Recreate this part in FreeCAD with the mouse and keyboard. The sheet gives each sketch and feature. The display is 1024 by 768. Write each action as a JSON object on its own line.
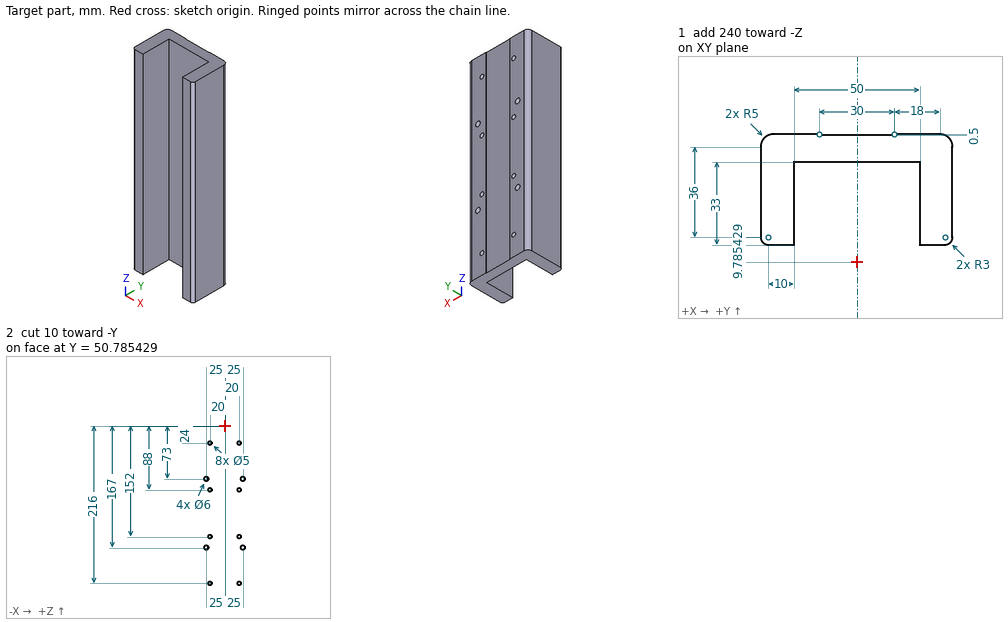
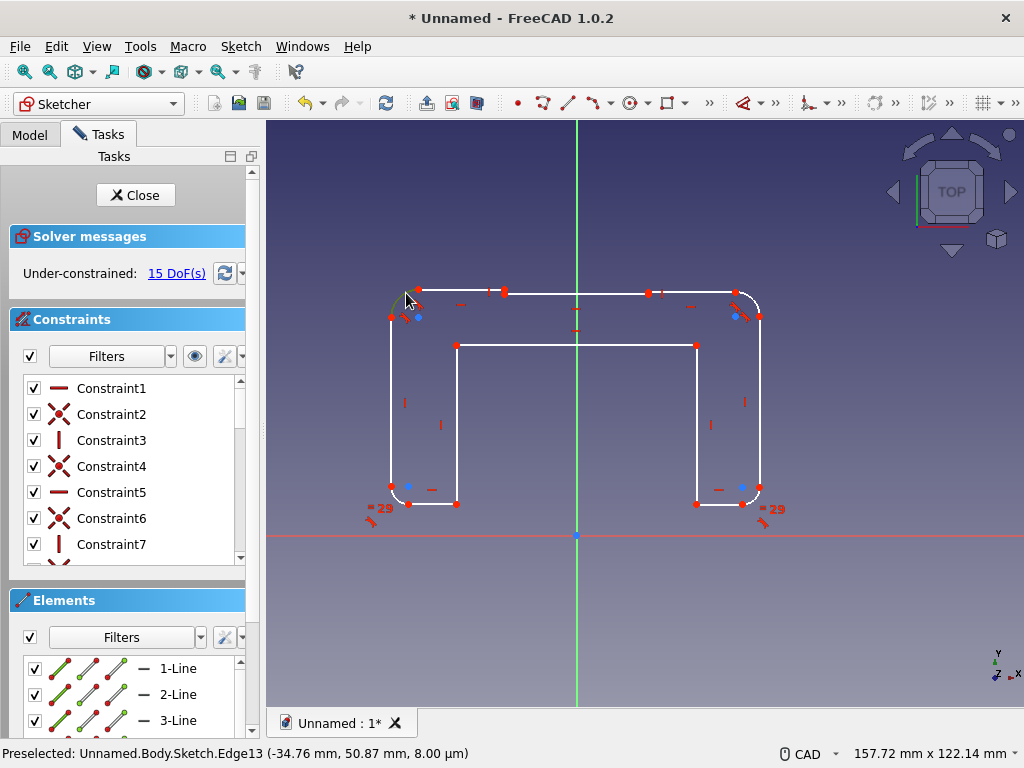
{"action": "left_click", "coordinate": [757, 305]}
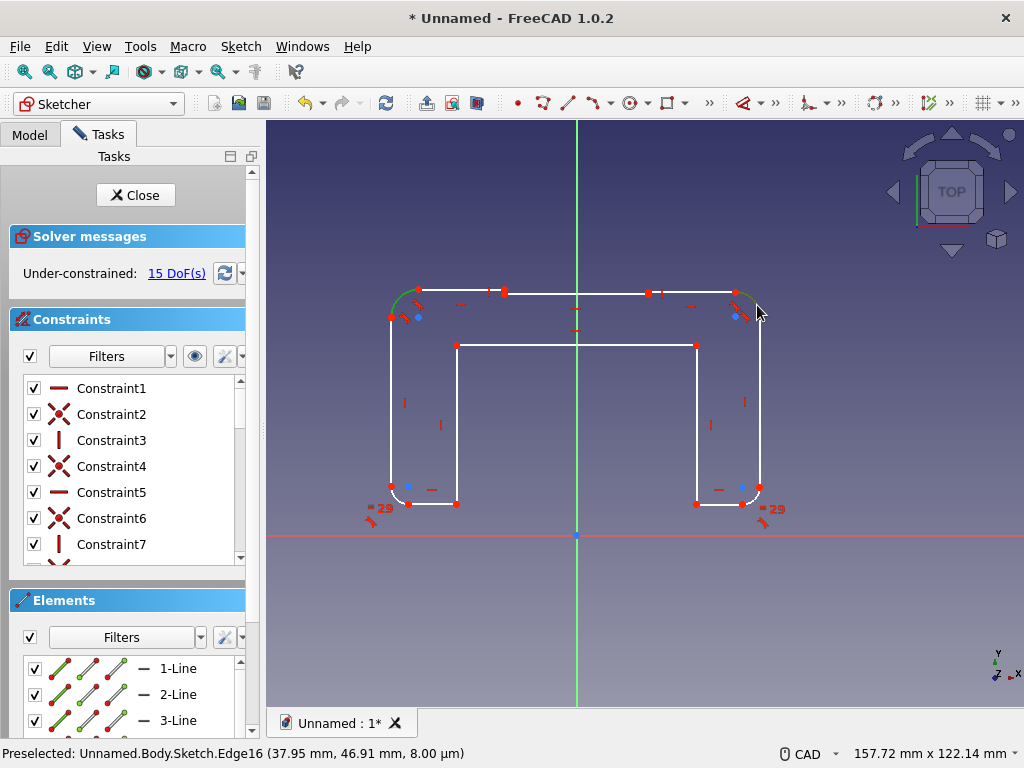
{"action": "key", "text": "e"}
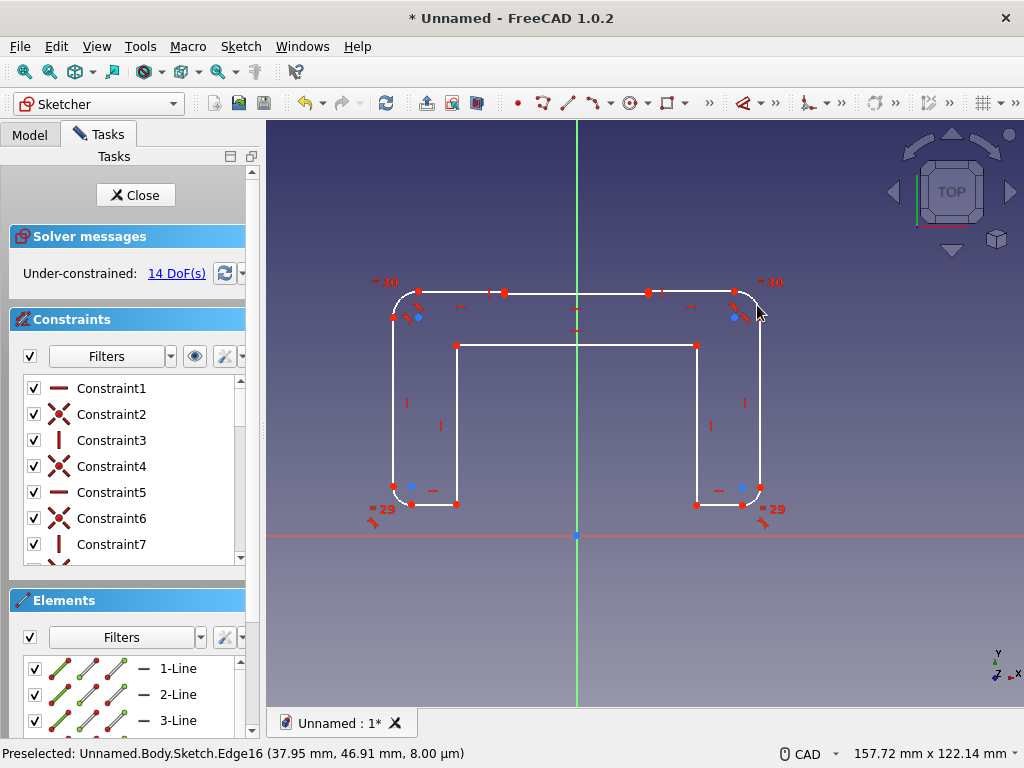
{"action": "left_click", "coordinate": [411, 487]}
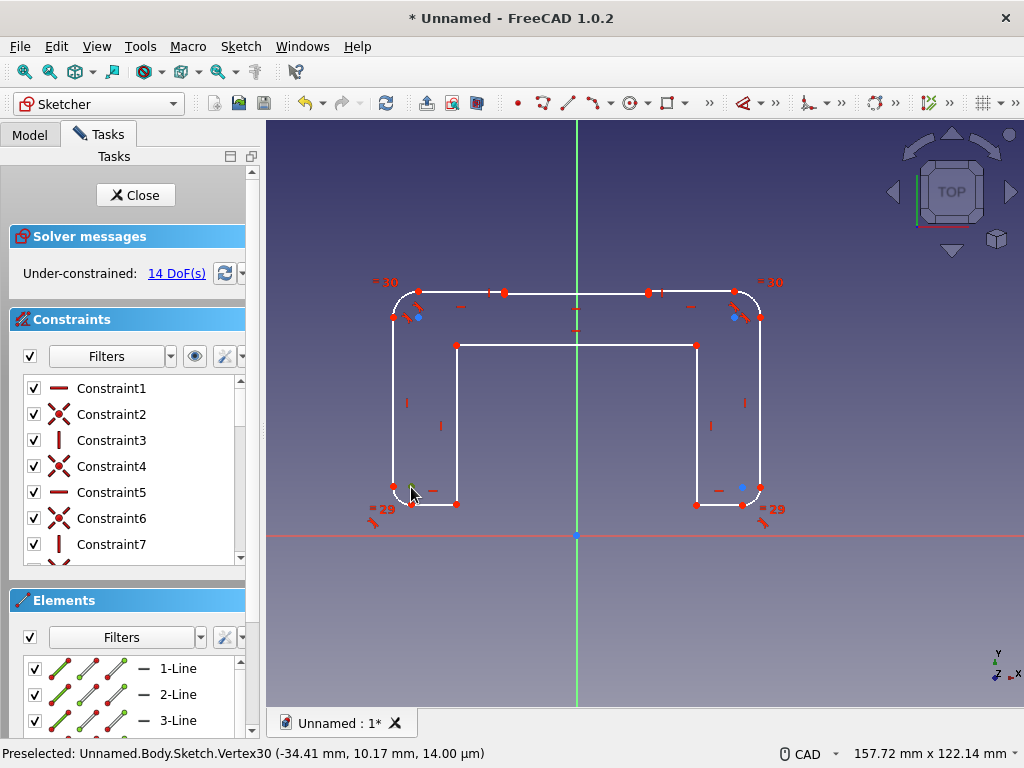
{"action": "left_click", "coordinate": [742, 487]}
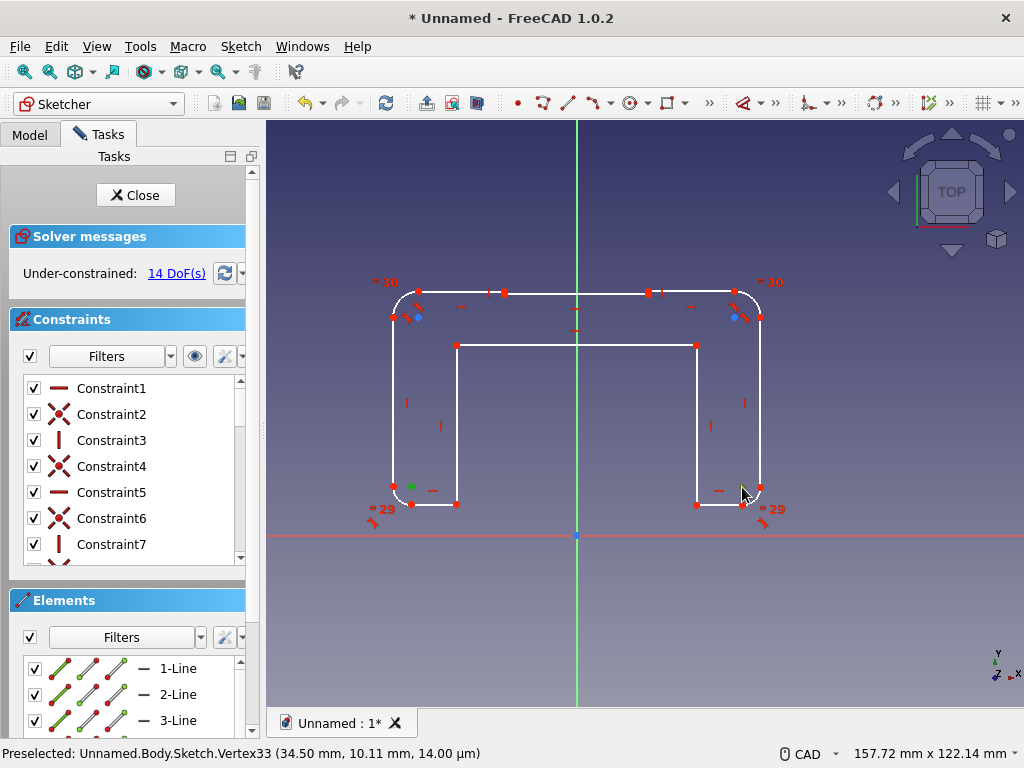
{"action": "left_click", "coordinate": [577, 641]}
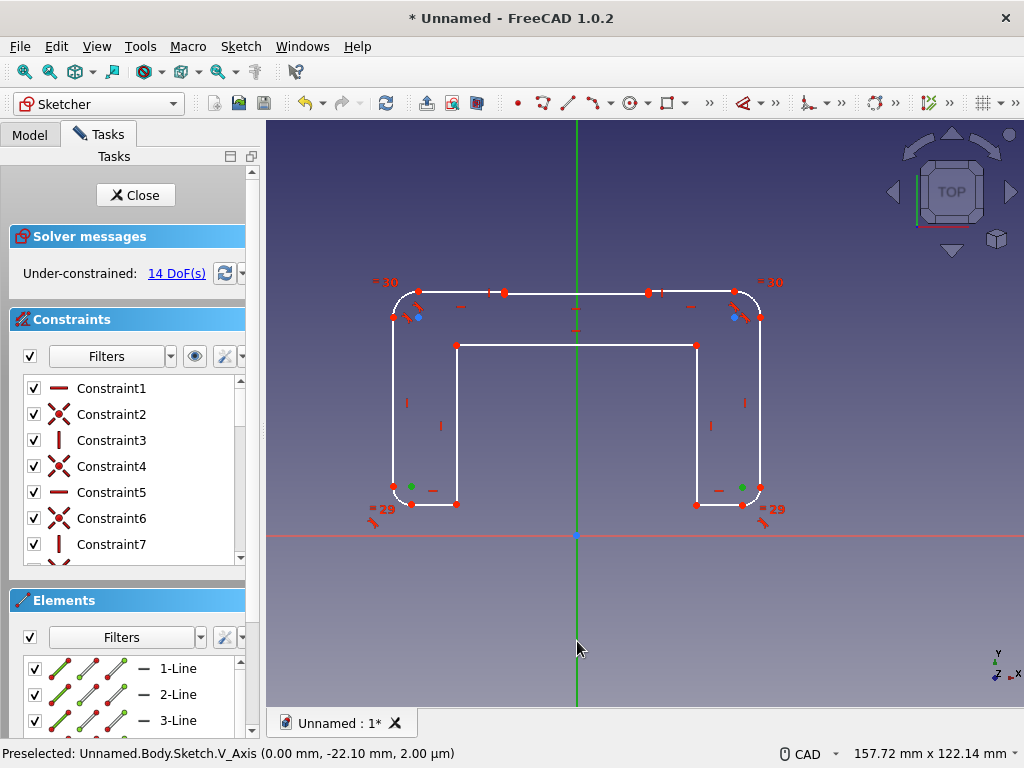
{"action": "key", "text": "s"}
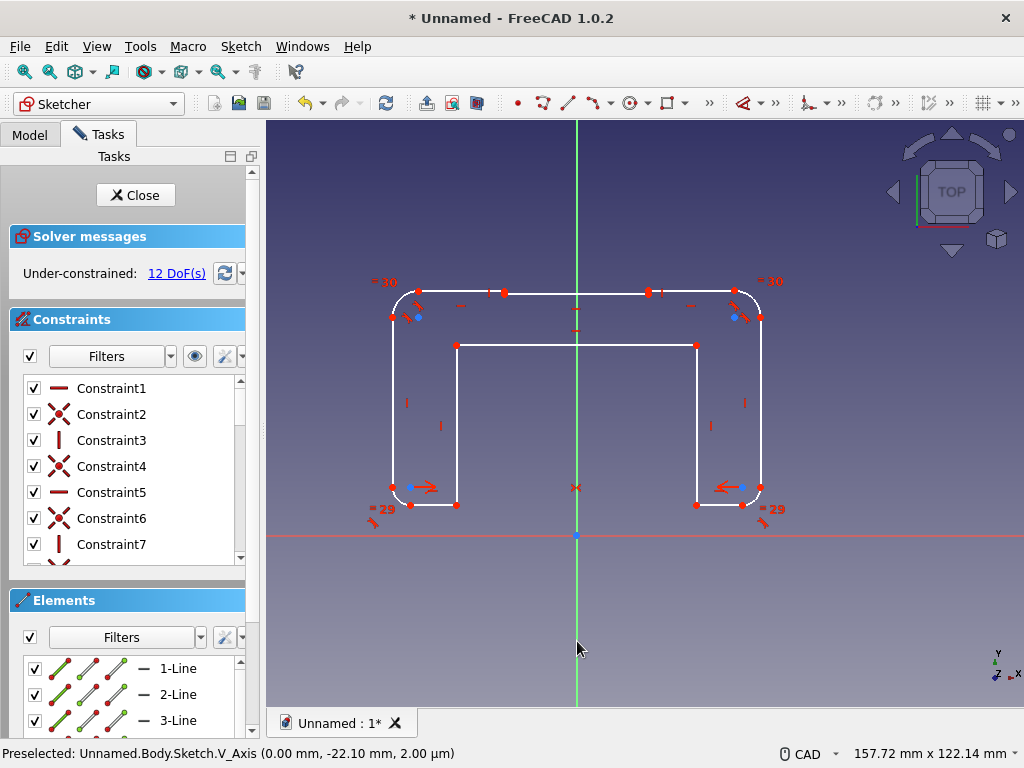
{"action": "scroll", "coordinate": [648, 291], "scroll_direction": "up", "scroll_amount": 7}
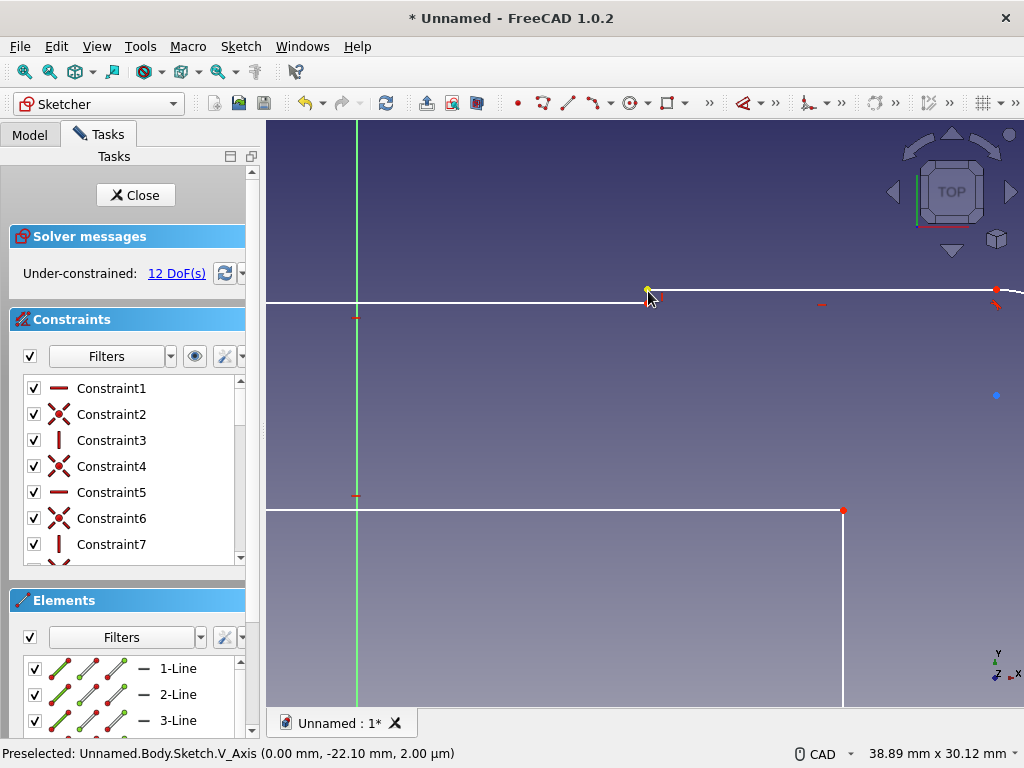
{"action": "left_click", "coordinate": [648, 290]}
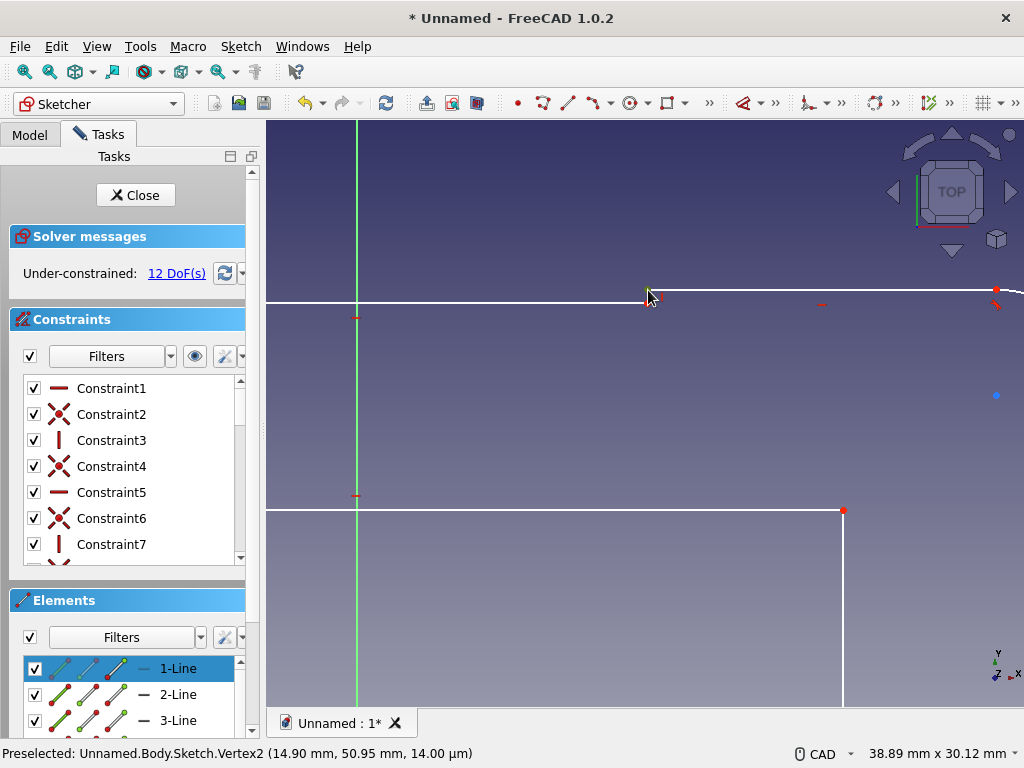
{"action": "scroll", "coordinate": [648, 291], "scroll_direction": "down", "scroll_amount": 7}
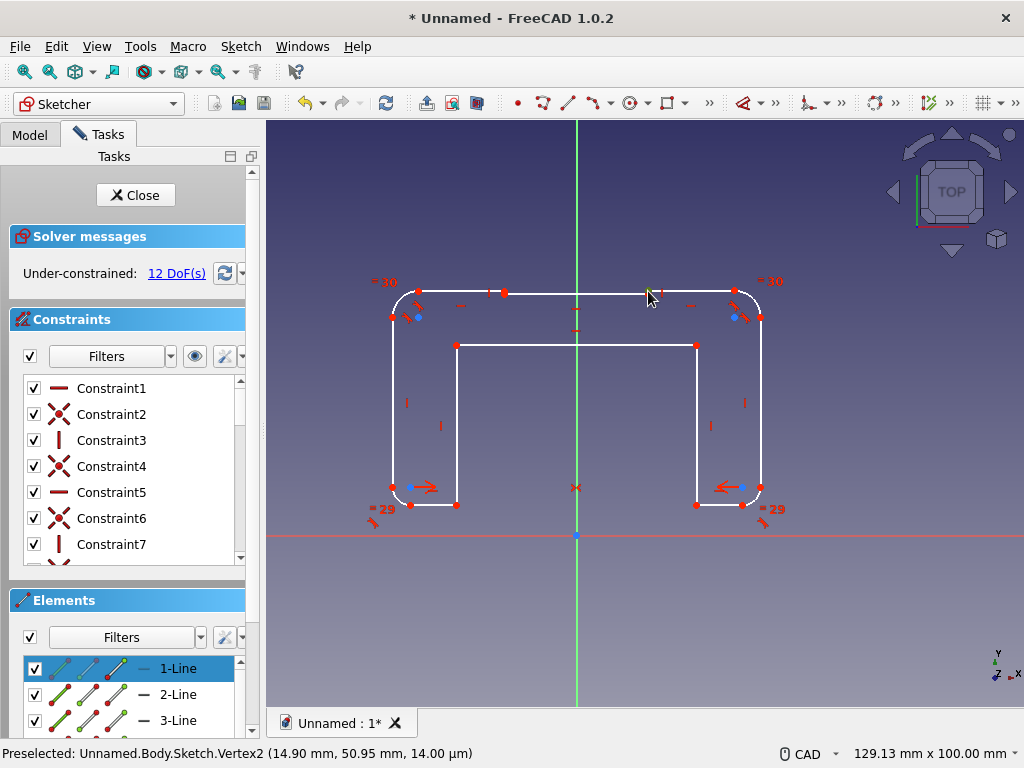
{"action": "scroll", "coordinate": [505, 291], "scroll_direction": "up", "scroll_amount": 7}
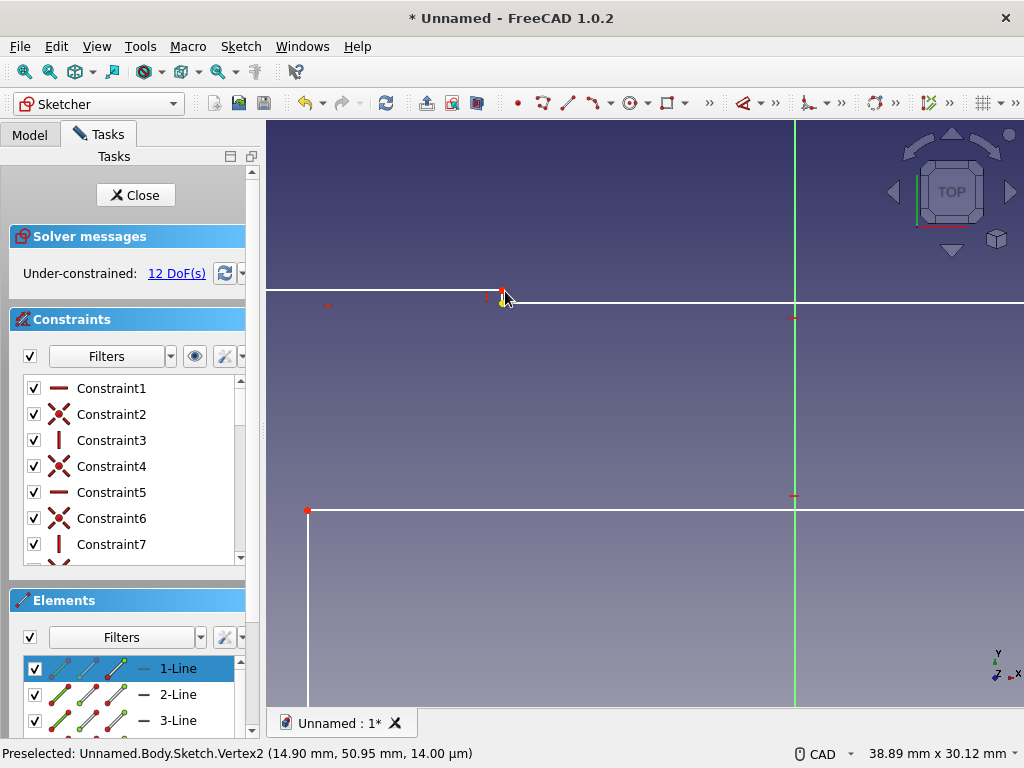
{"action": "left_click", "coordinate": [502, 290]}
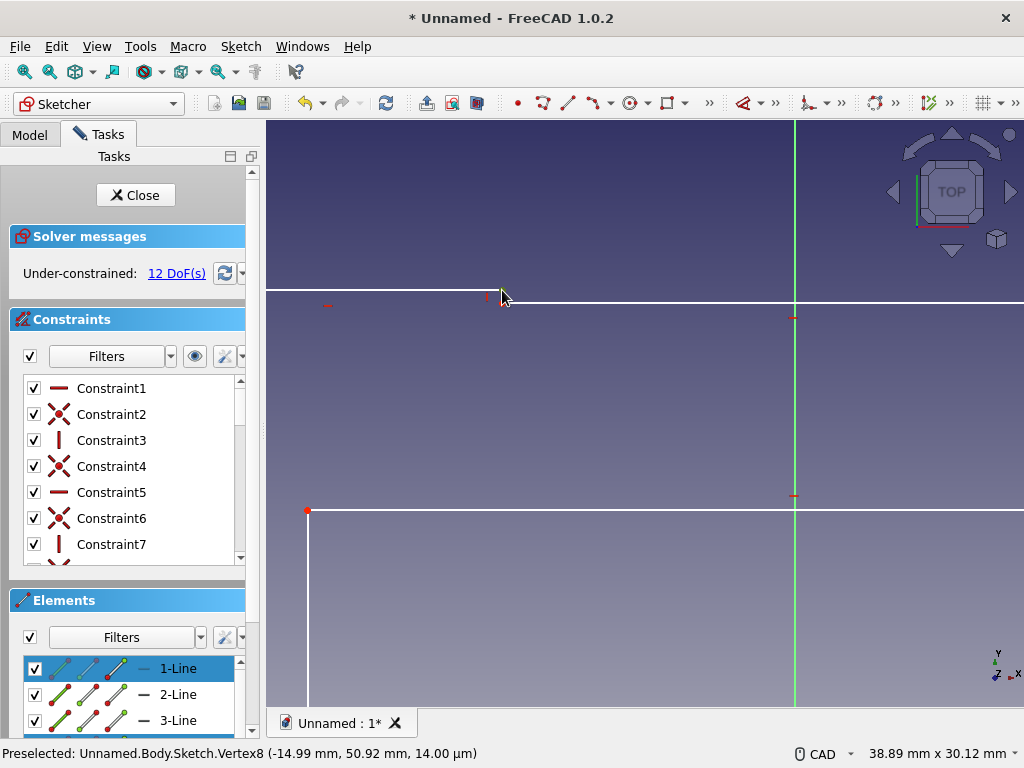
{"action": "left_click", "coordinate": [795, 641]}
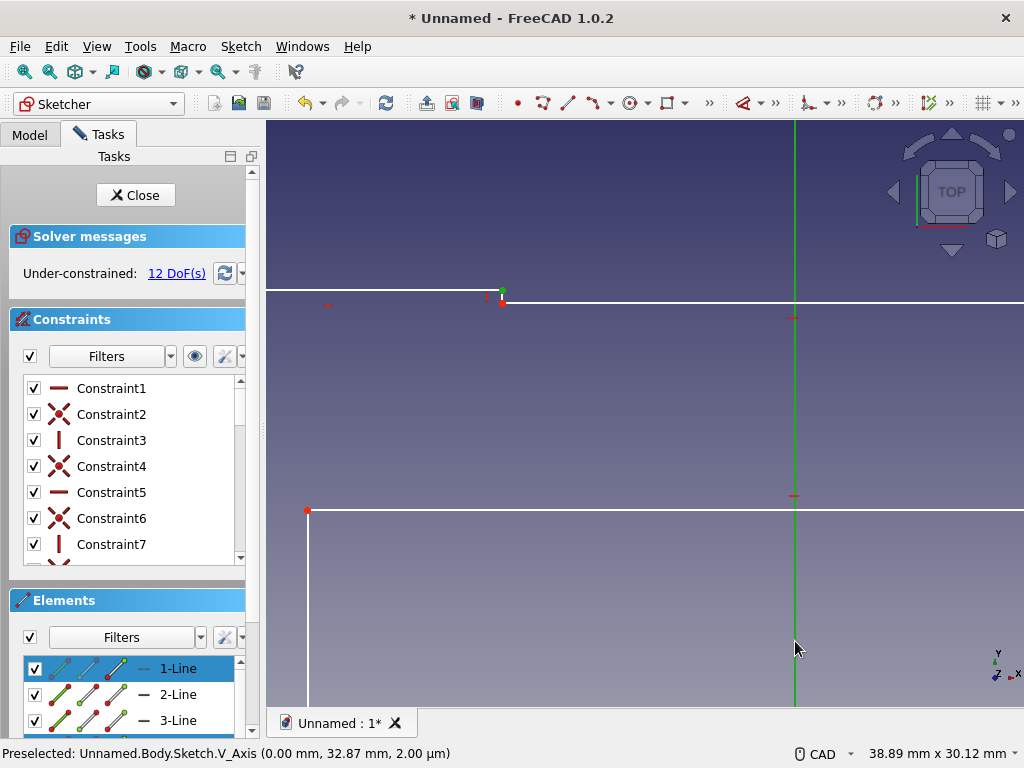
{"action": "key", "text": "s"}